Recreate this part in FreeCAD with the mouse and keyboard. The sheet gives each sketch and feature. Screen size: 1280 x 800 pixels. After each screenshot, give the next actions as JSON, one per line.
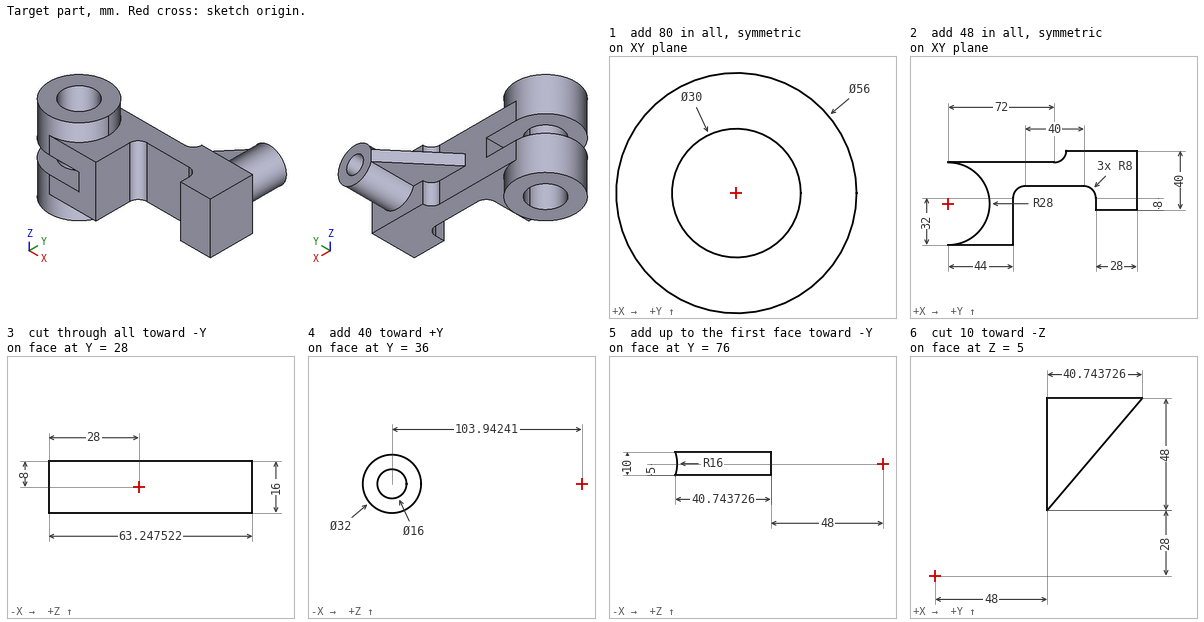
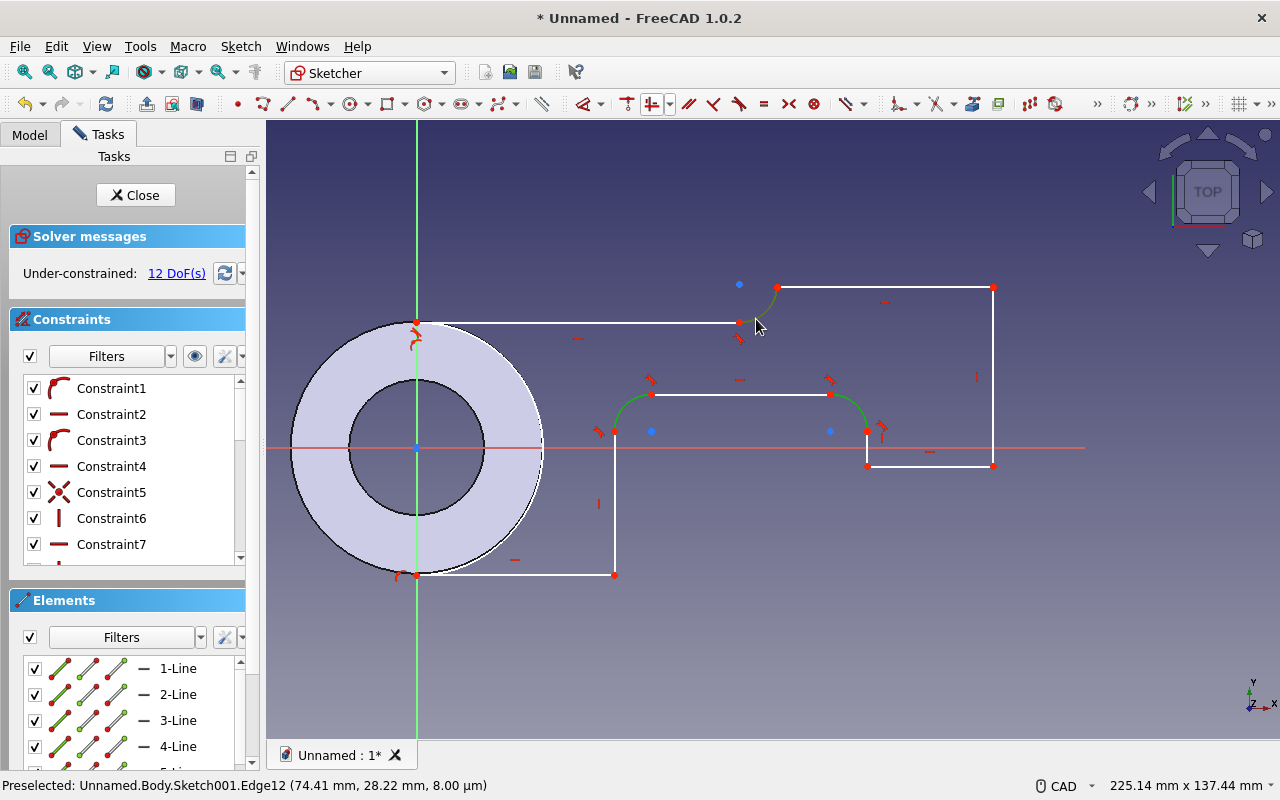
{"action": "left_click", "coordinate": [764, 104]}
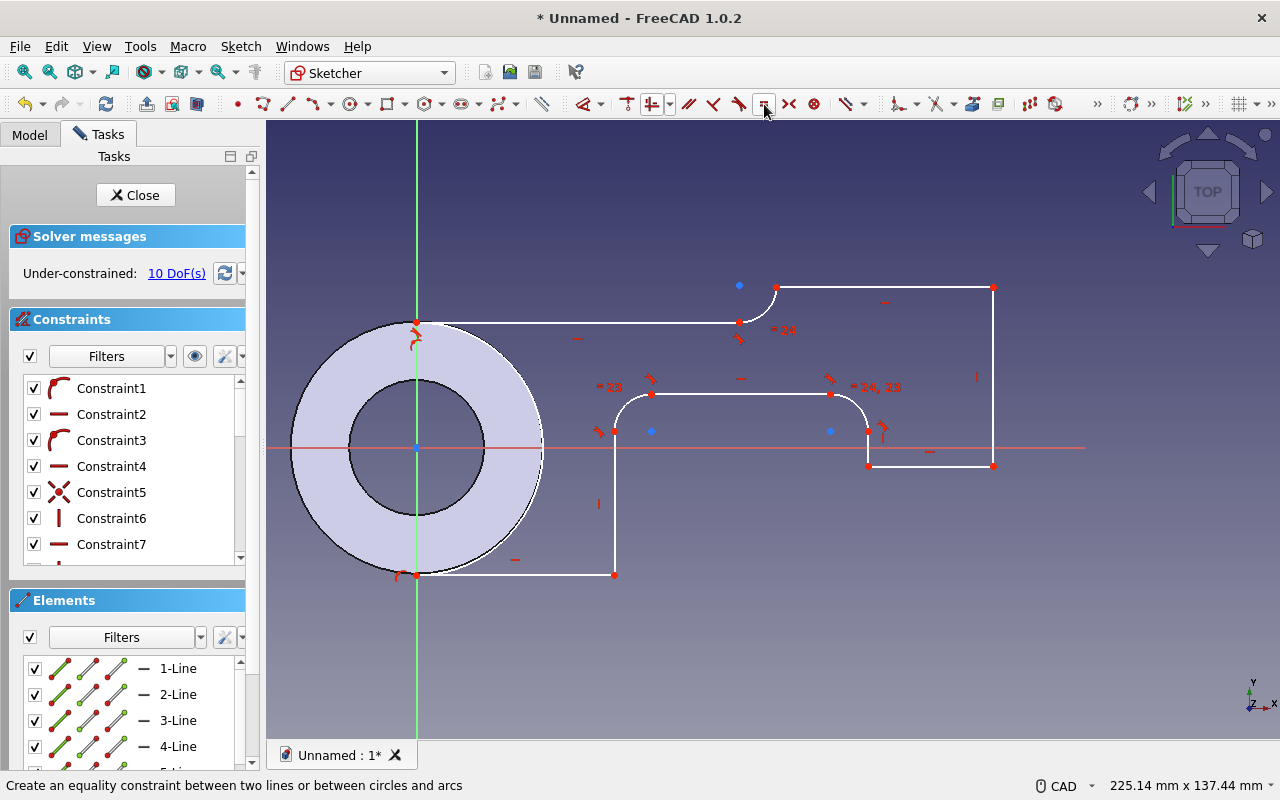
{"action": "left_click", "coordinate": [417, 449]}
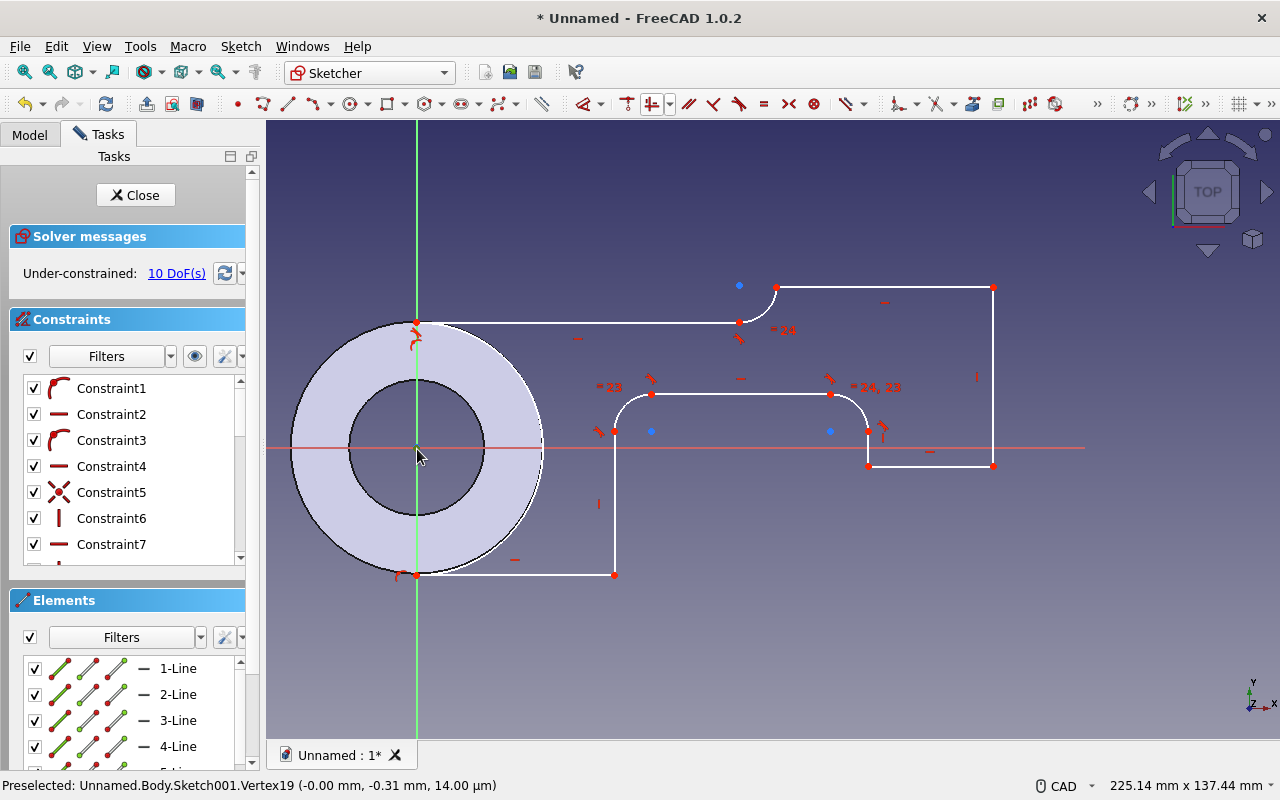
{"action": "left_click", "coordinate": [353, 448]}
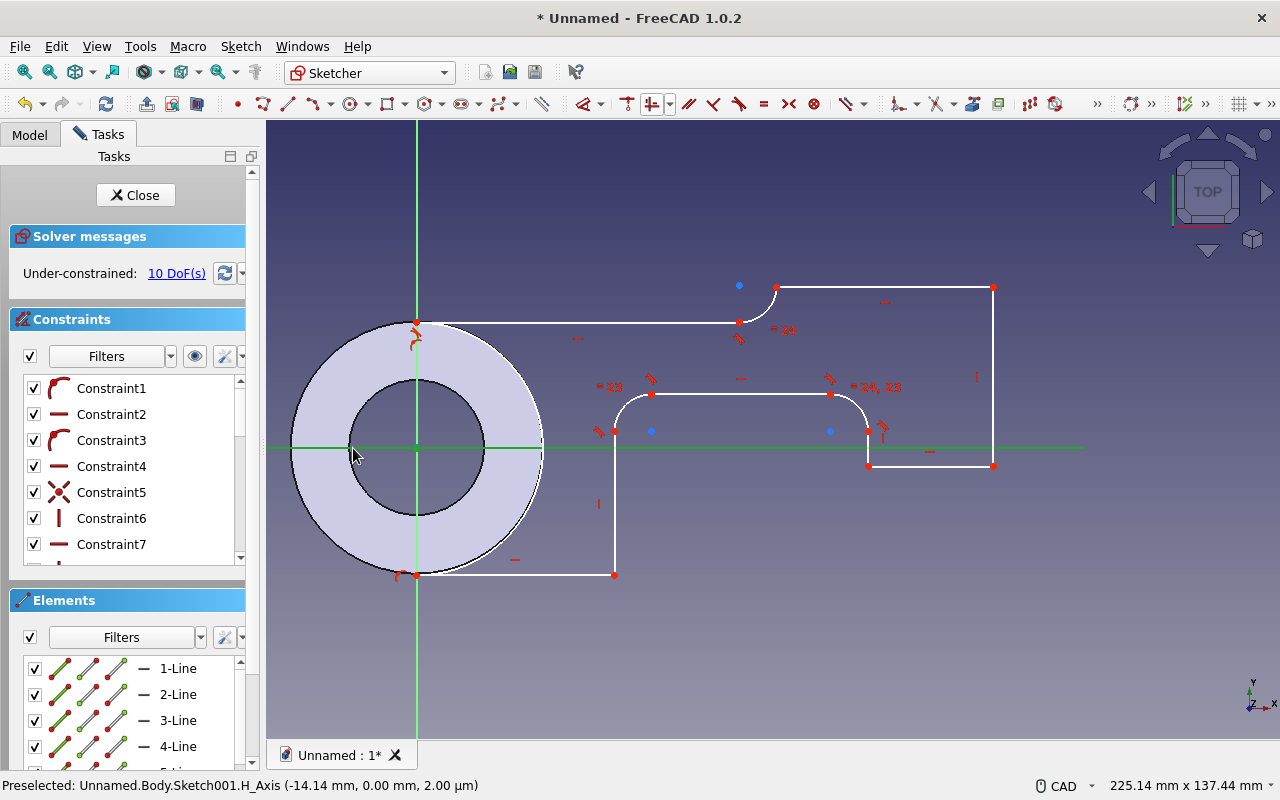
{"action": "left_click", "coordinate": [627, 104]}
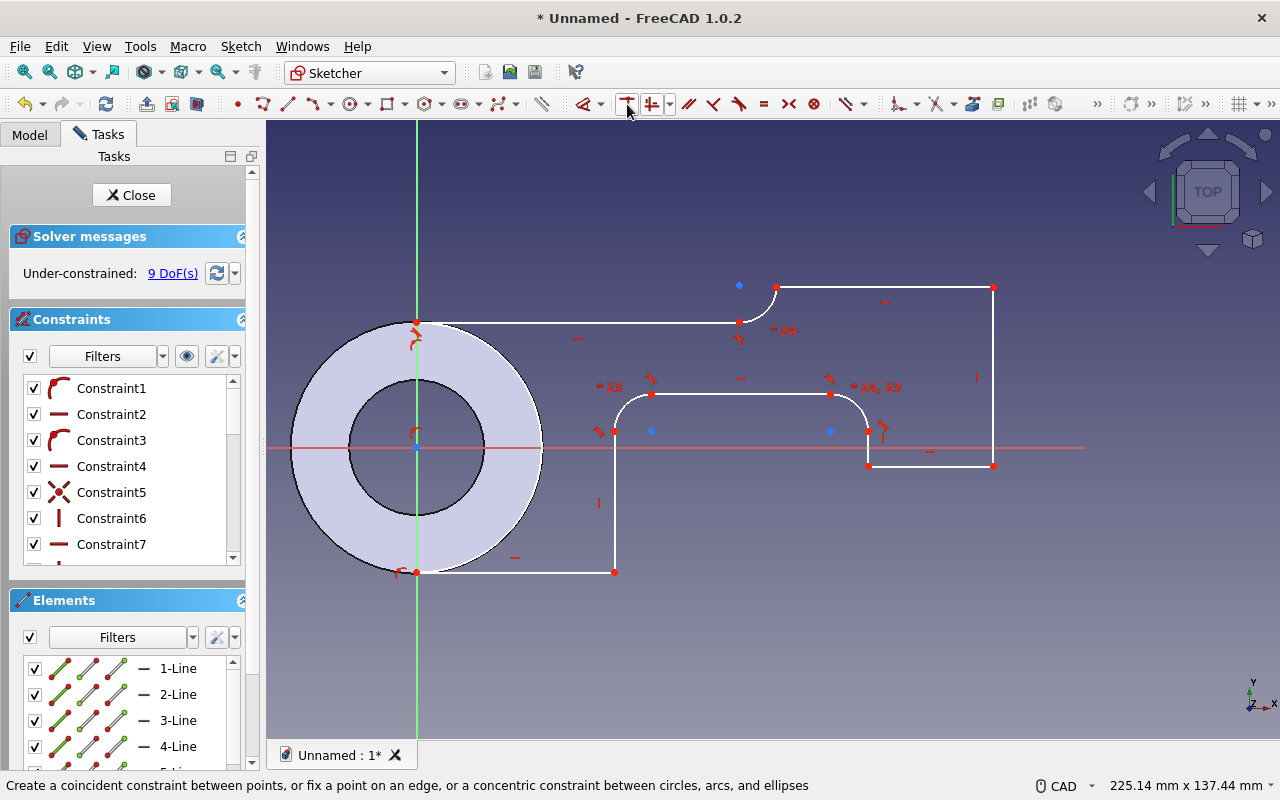
{"action": "left_click", "coordinate": [582, 104]}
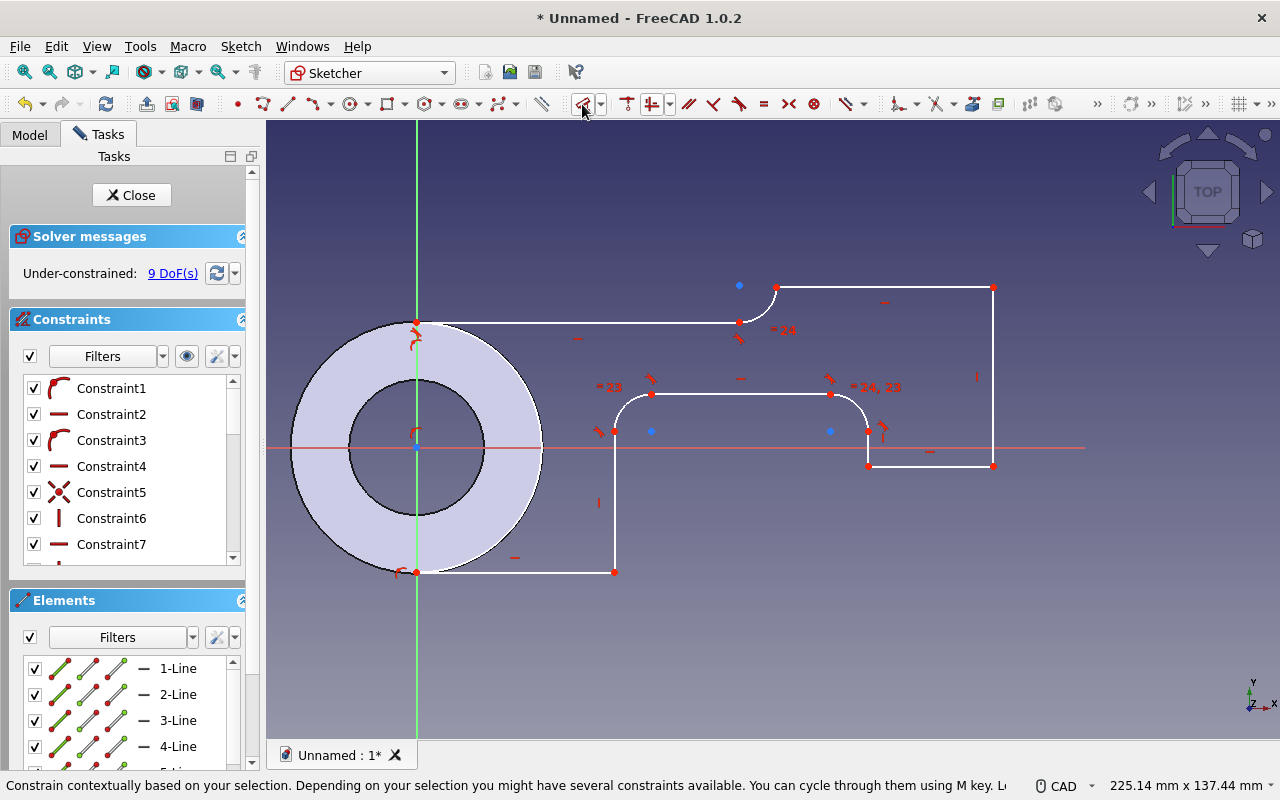
{"action": "left_click", "coordinate": [518, 521]}
{"action": "left_click", "coordinate": [544, 540]}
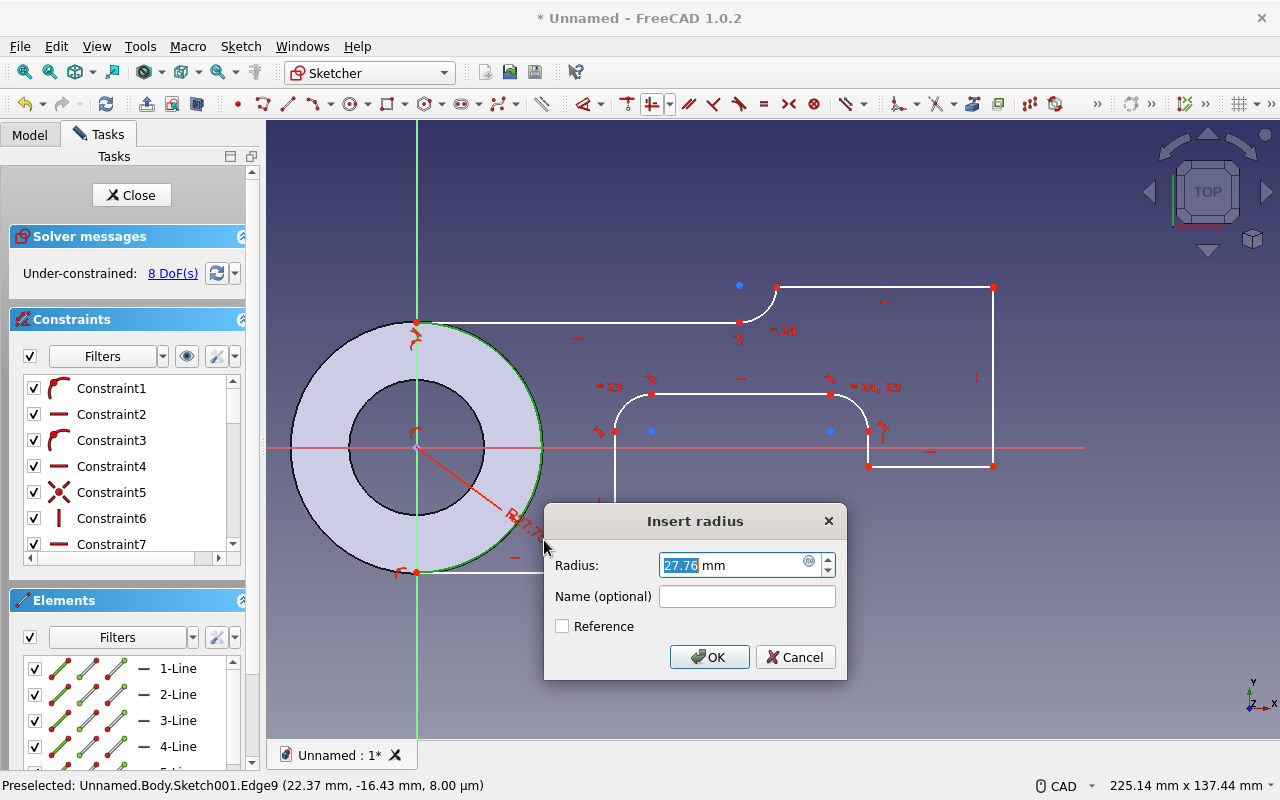
{"action": "type", "text": "28"}
{"action": "key", "text": "Return"}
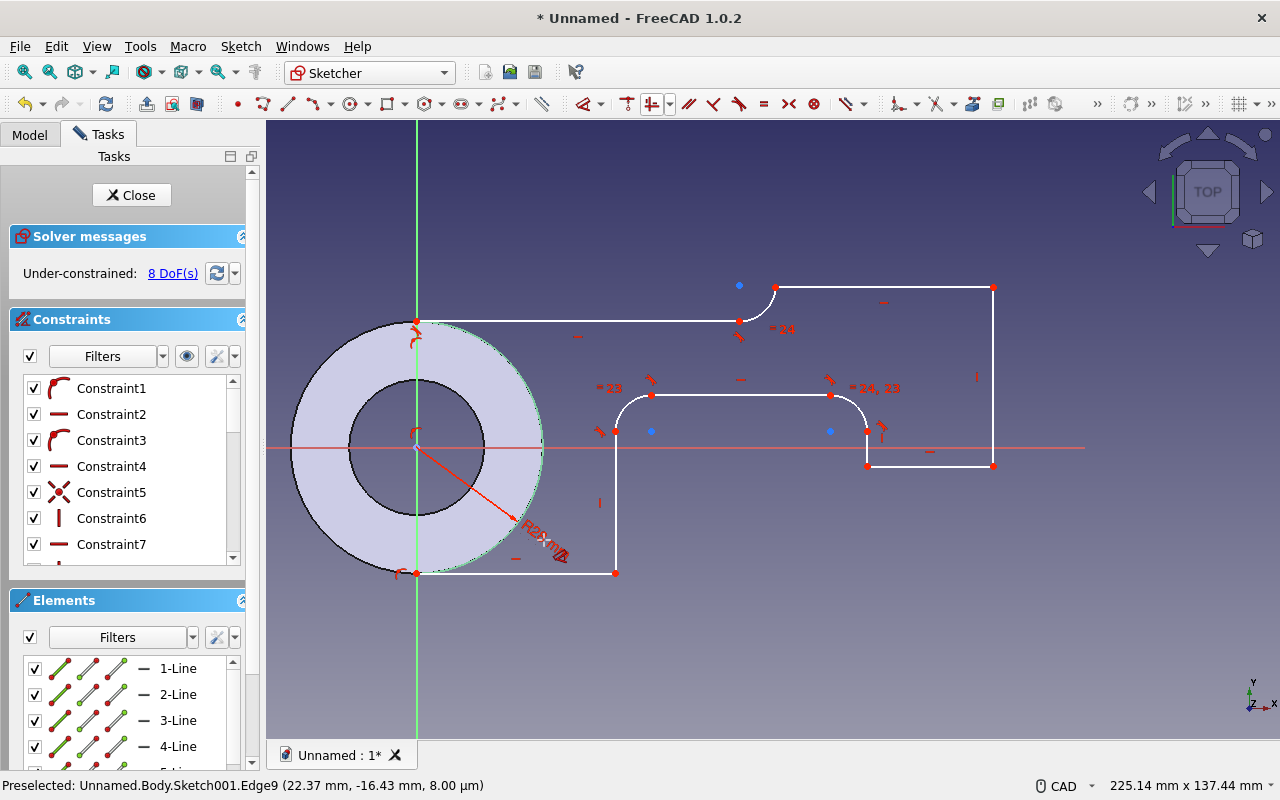
{"action": "left_click", "coordinate": [635, 399]}
{"action": "left_click", "coordinate": [620, 371]}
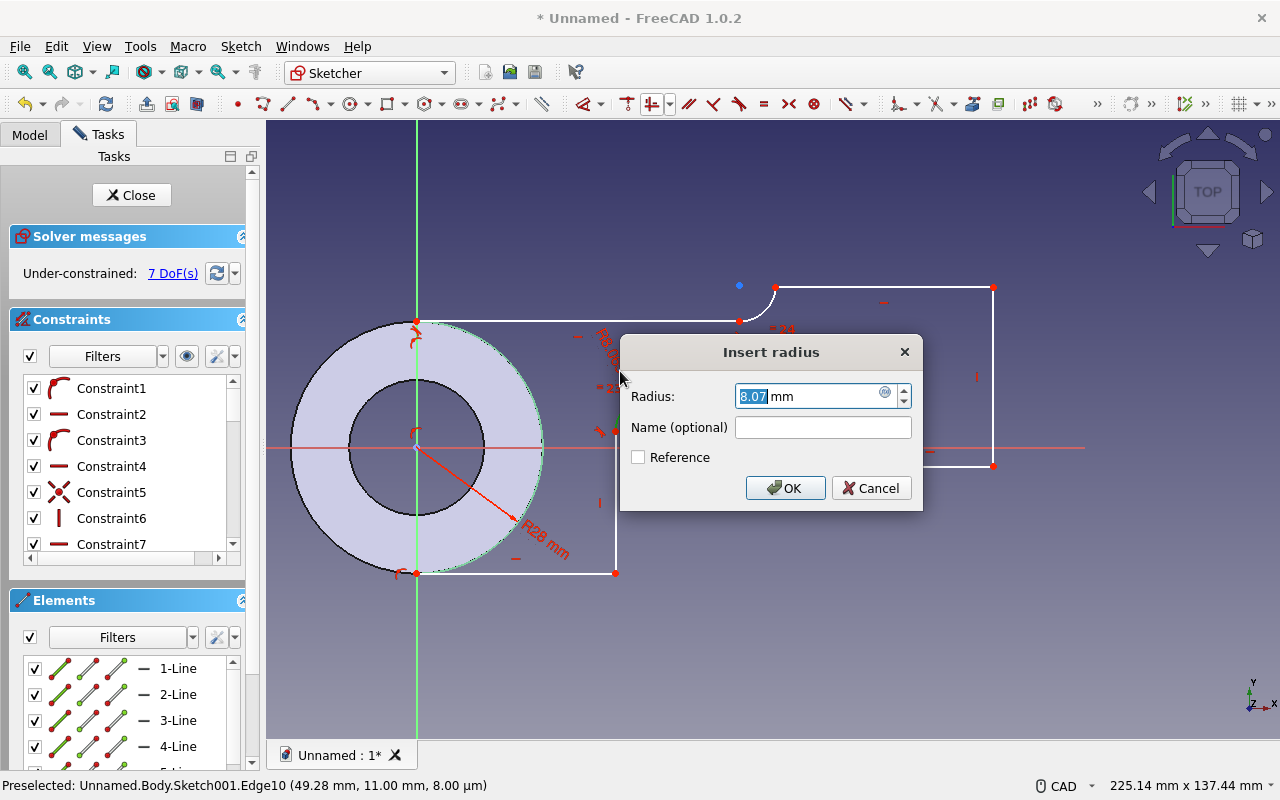
{"action": "type", "text": "8"}
{"action": "key", "text": "Return"}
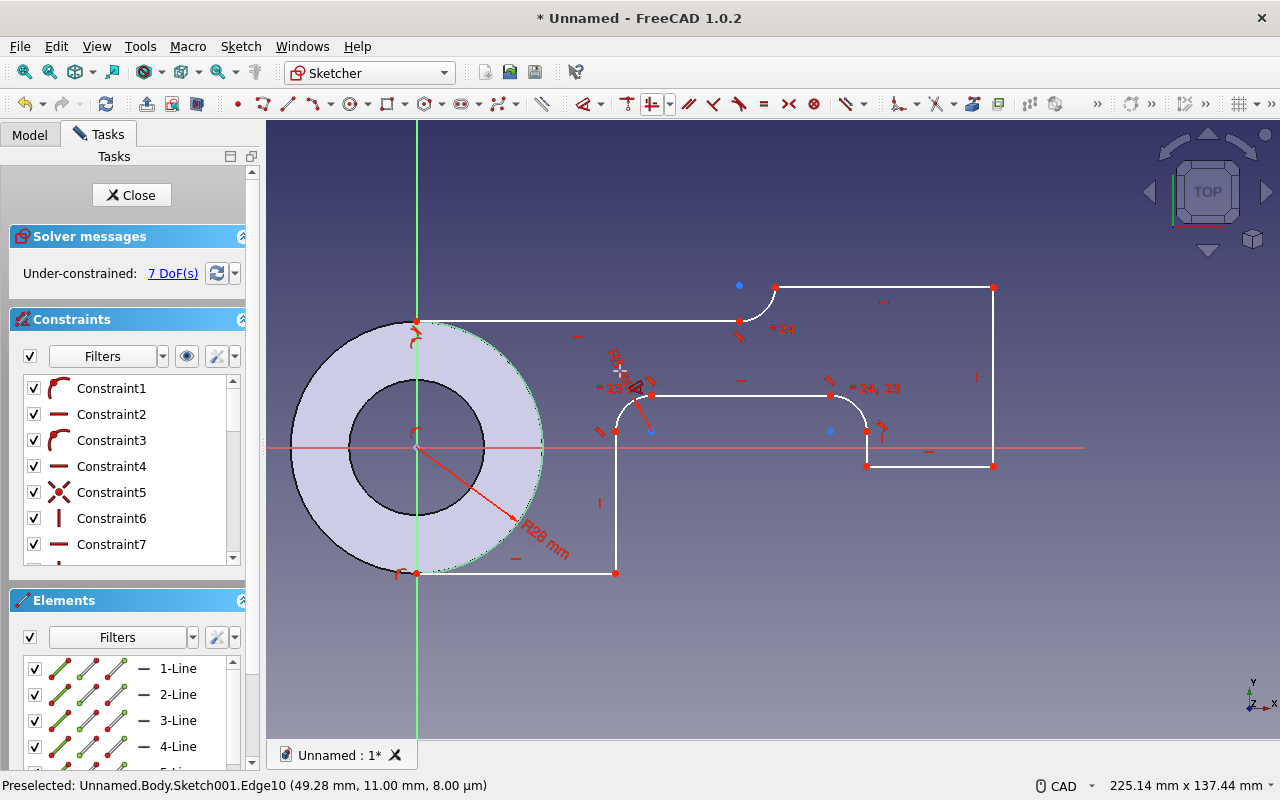
{"action": "left_click", "coordinate": [867, 446]}
{"action": "left_click", "coordinate": [833, 461]}